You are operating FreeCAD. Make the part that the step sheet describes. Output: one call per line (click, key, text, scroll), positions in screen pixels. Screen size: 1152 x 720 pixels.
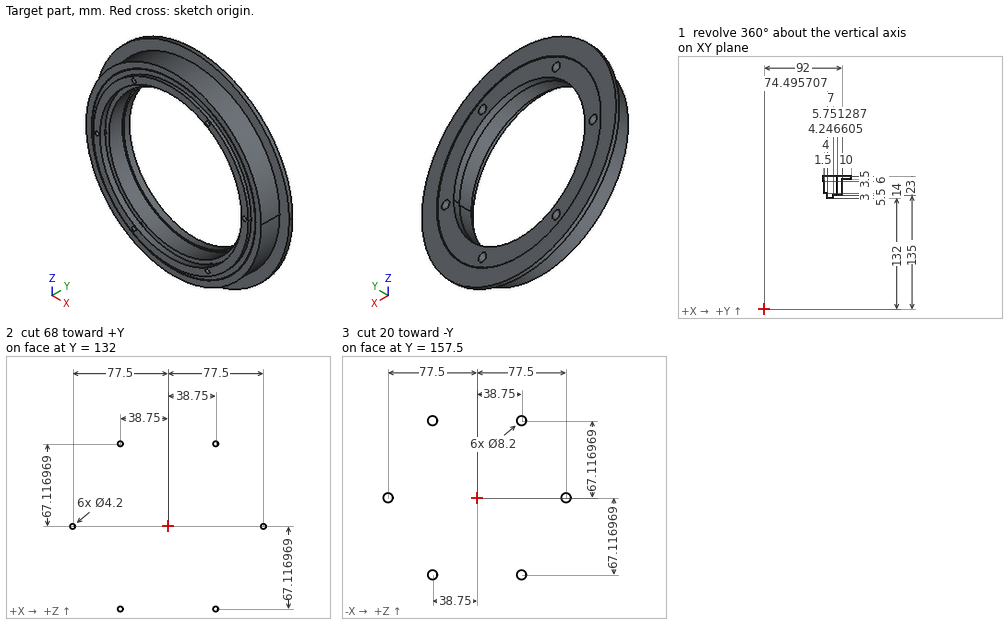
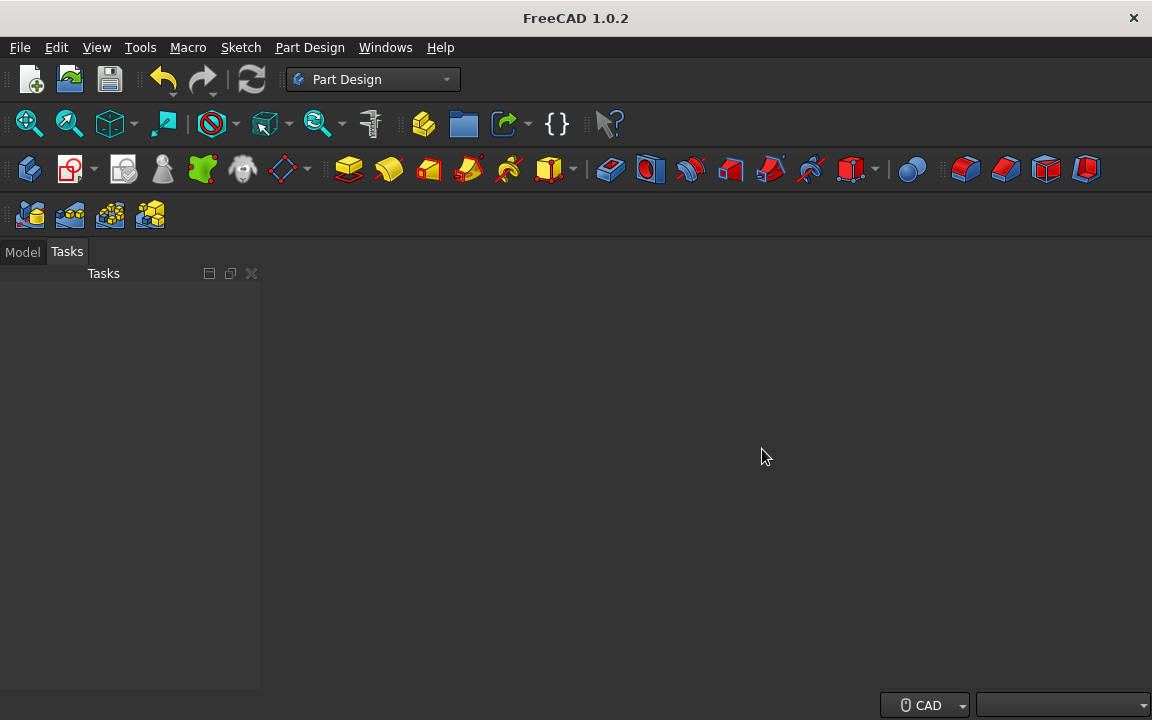
click(30, 80)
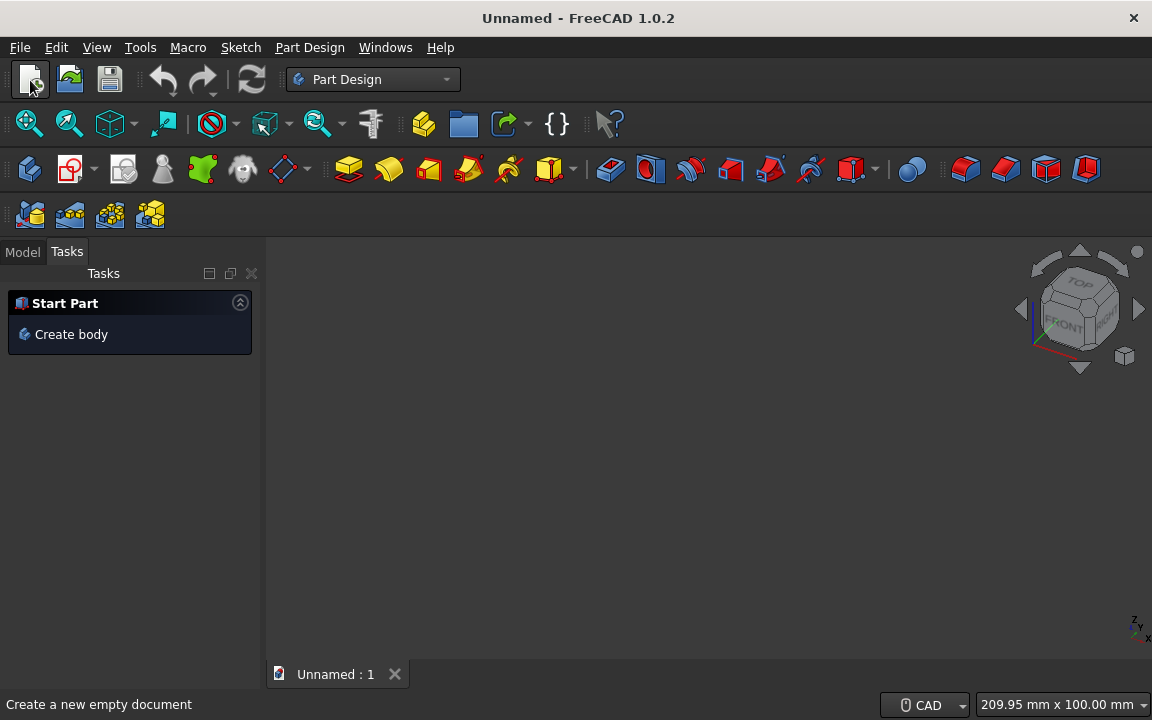
click(30, 170)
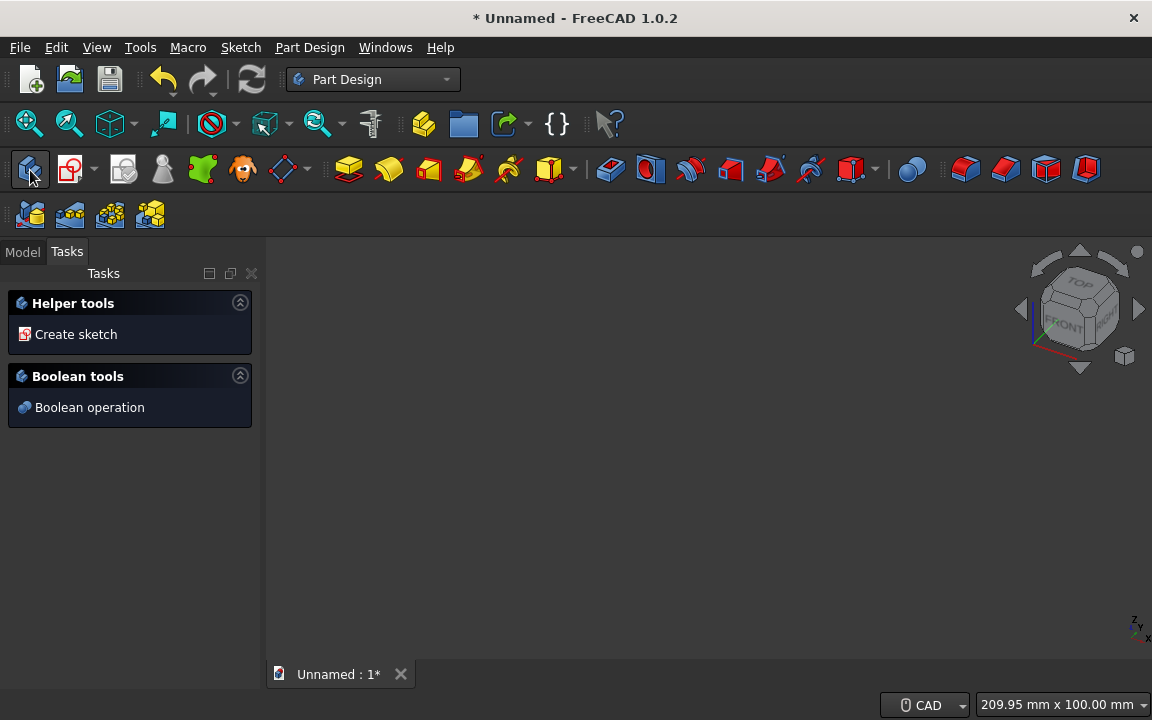
click(23, 251)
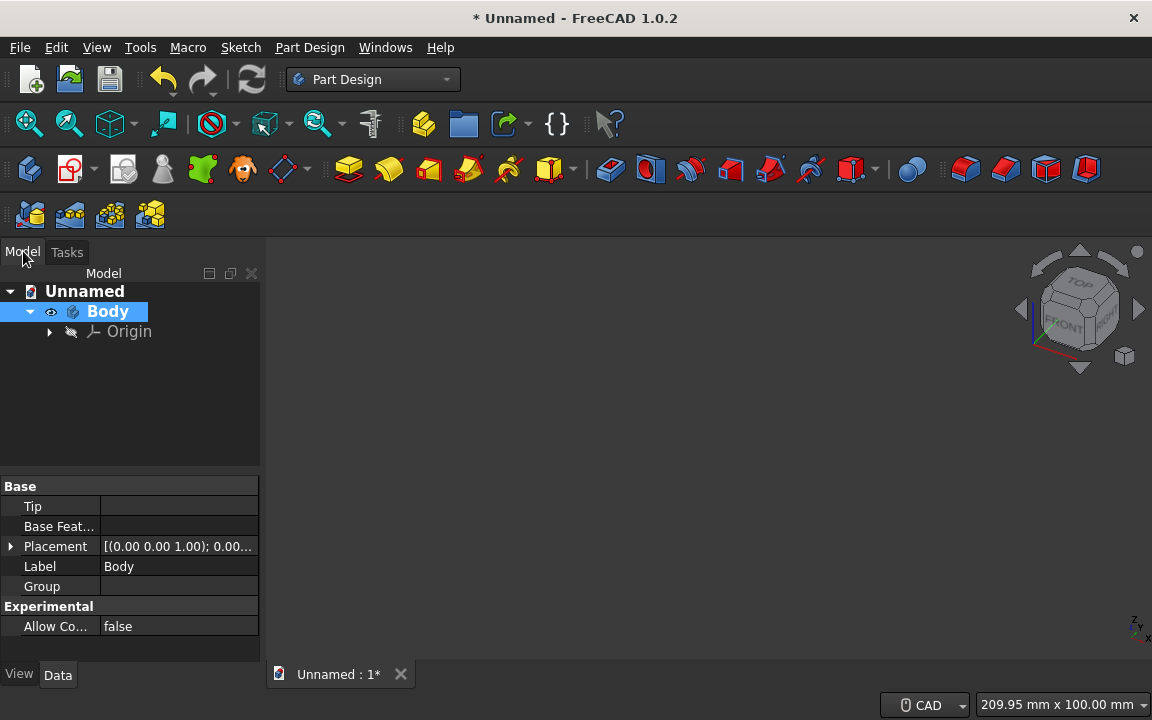
click(96, 312)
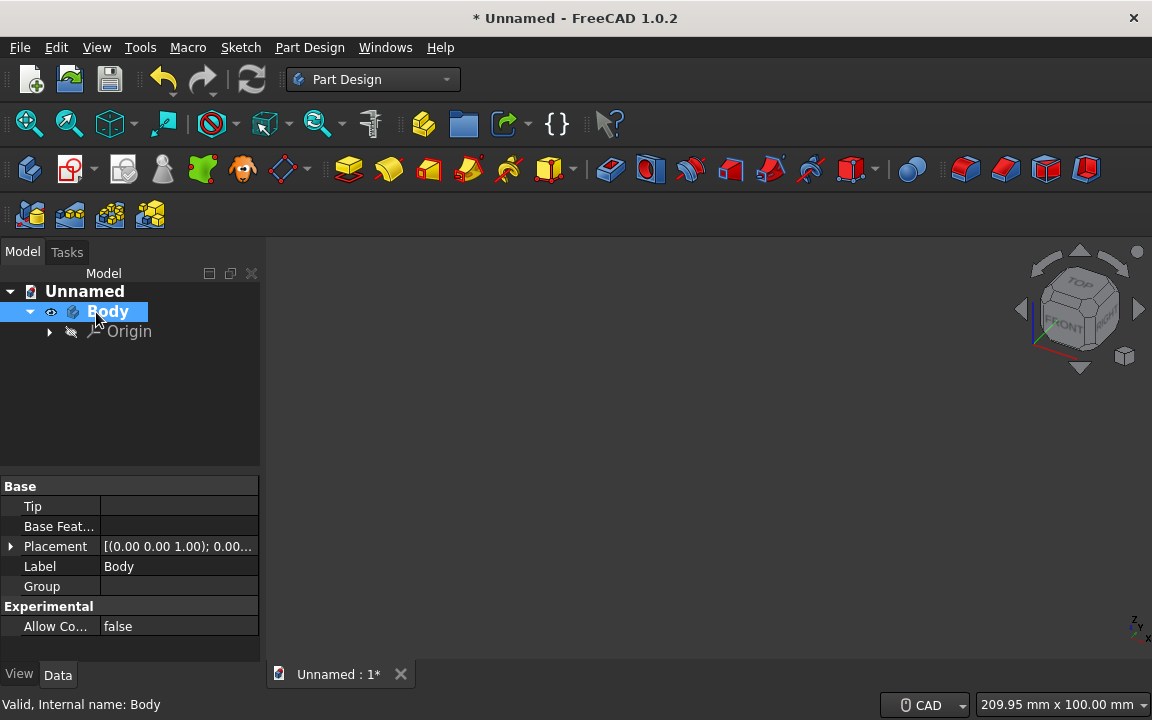
click(146, 626)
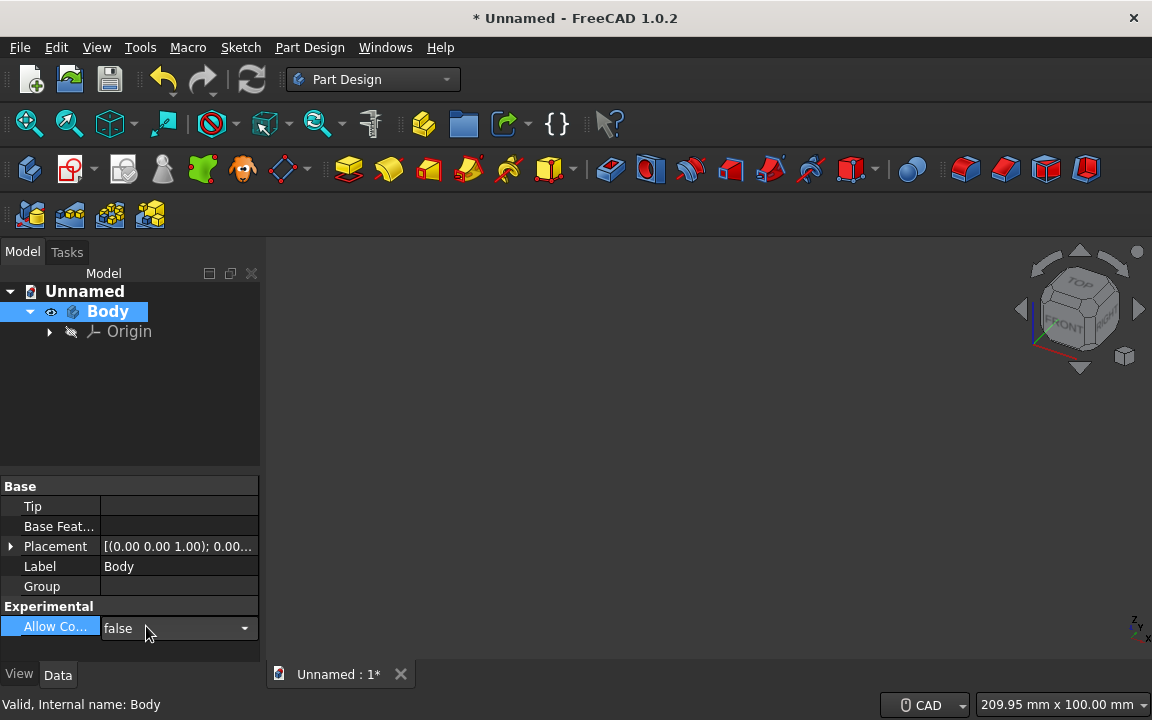
click(146, 626)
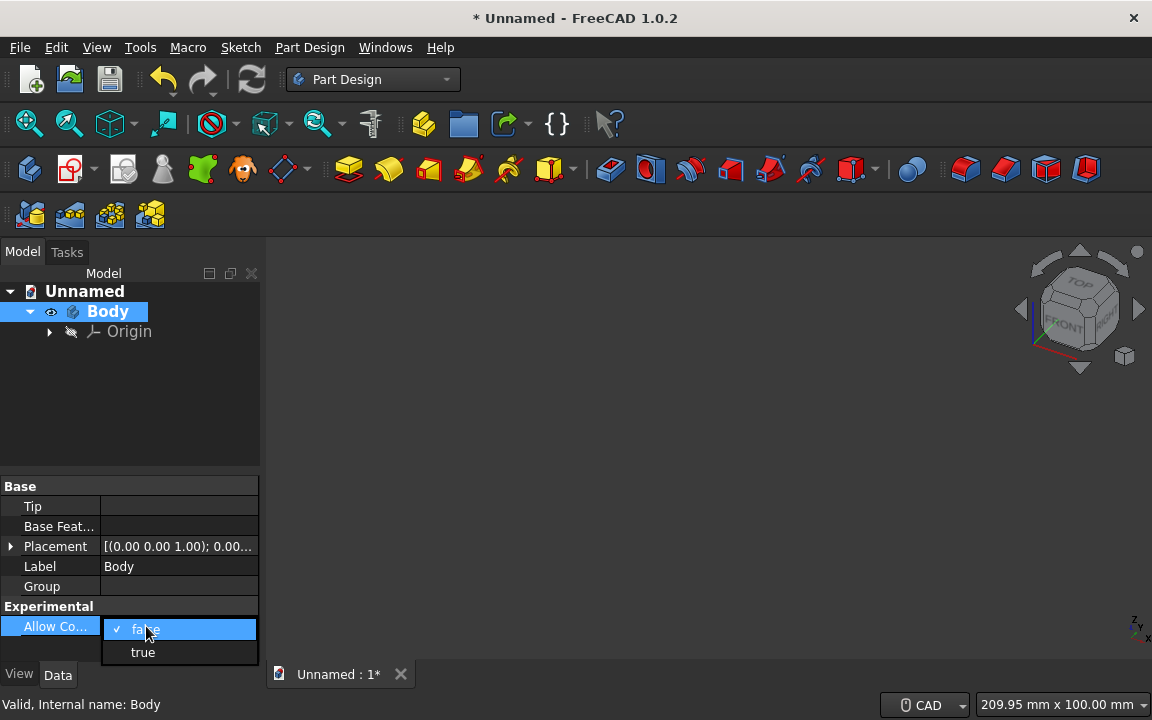
click(179, 652)
key(Return)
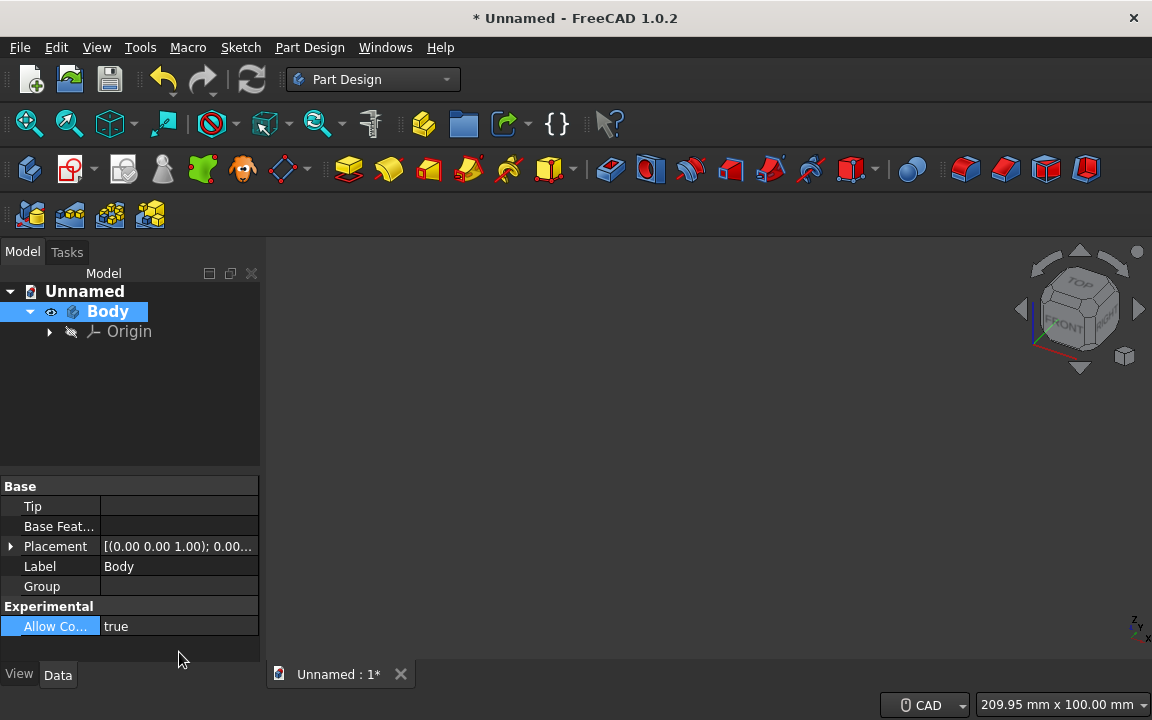
click(306, 619)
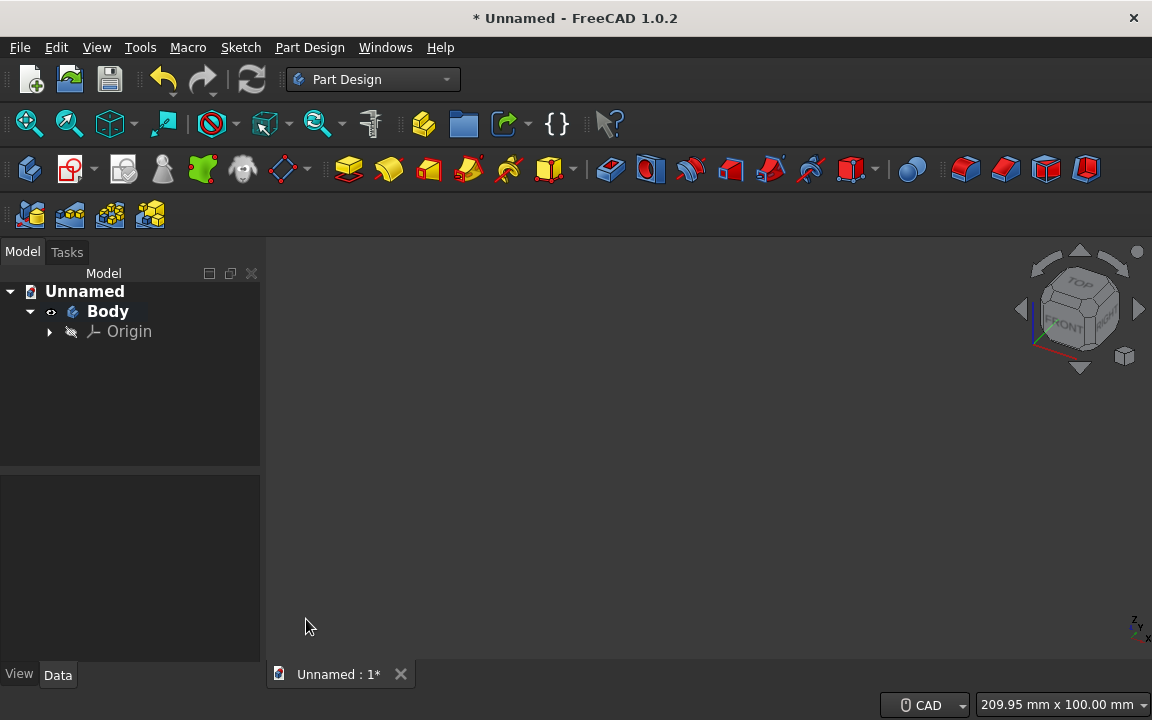
click(70, 170)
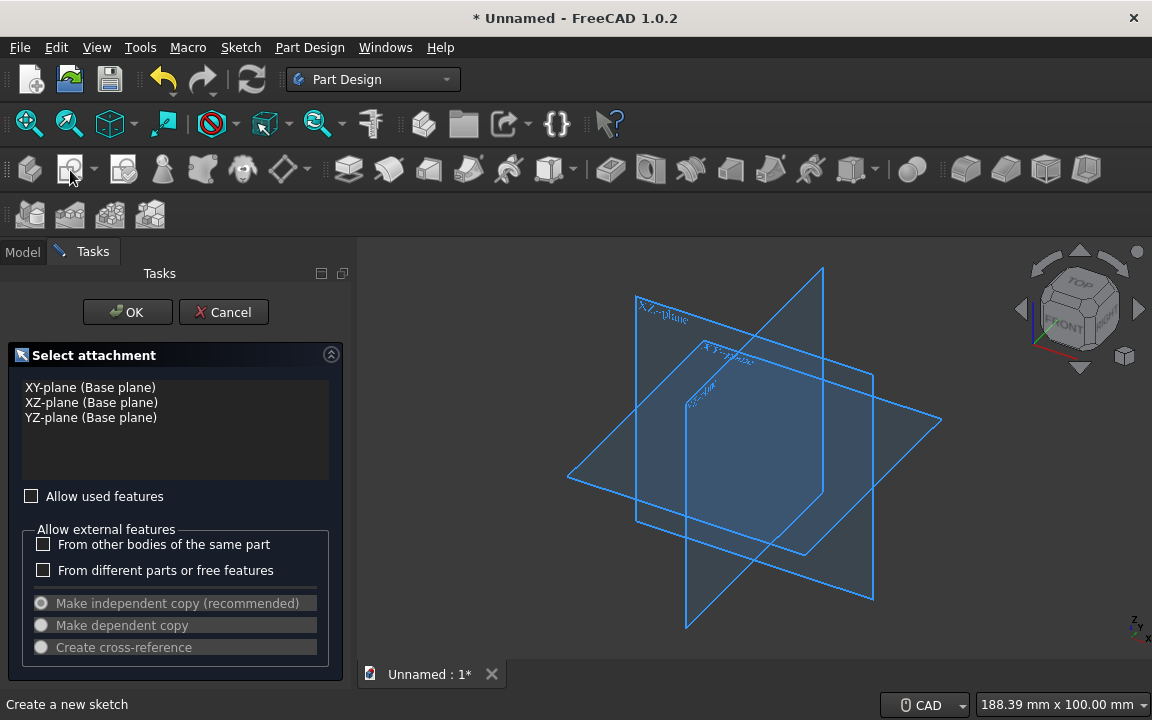
click(82, 388)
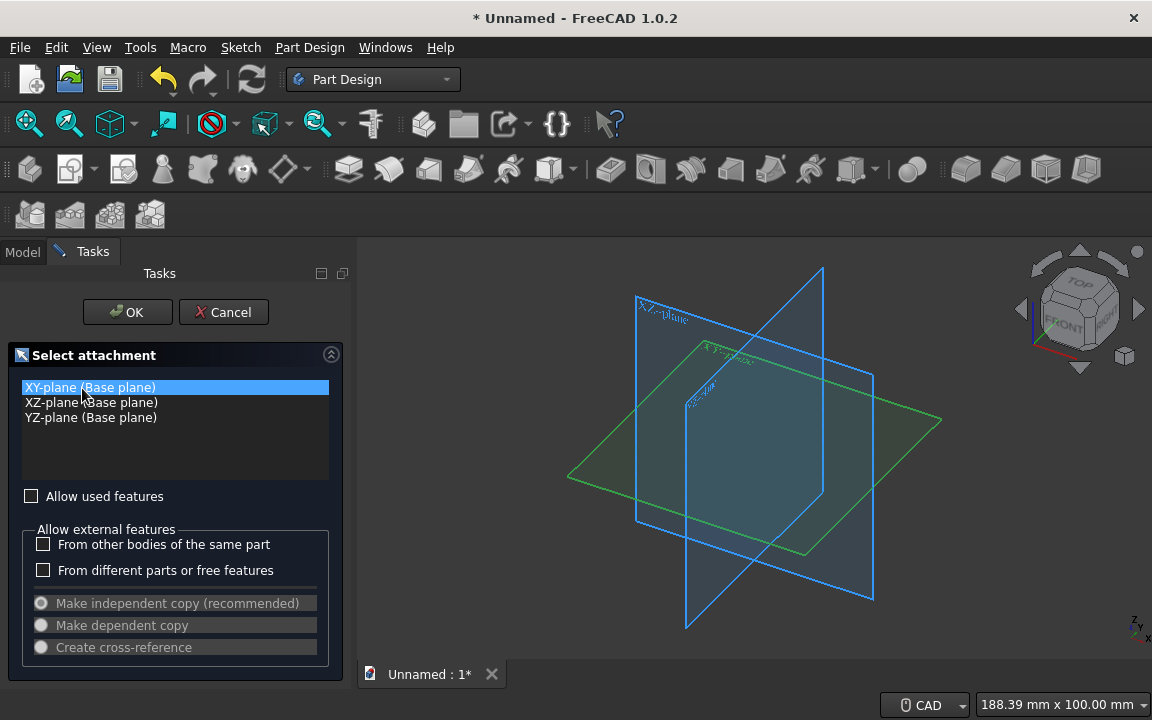
click(128, 312)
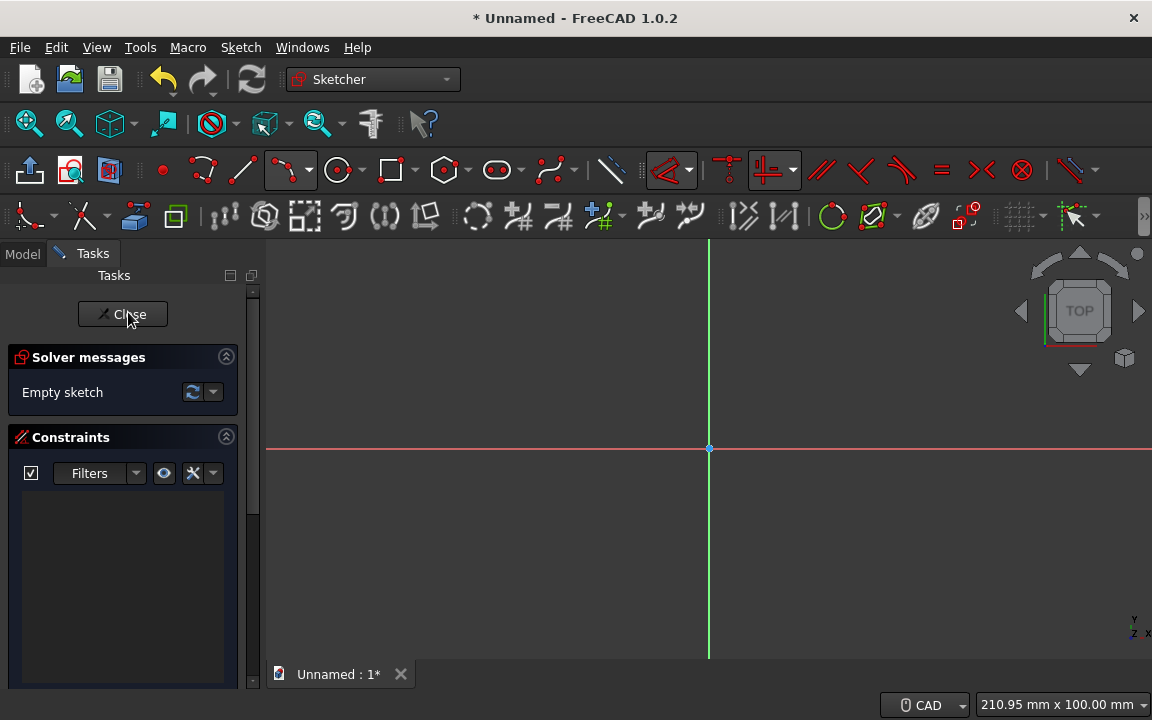
scroll(640, 449, down, 5)